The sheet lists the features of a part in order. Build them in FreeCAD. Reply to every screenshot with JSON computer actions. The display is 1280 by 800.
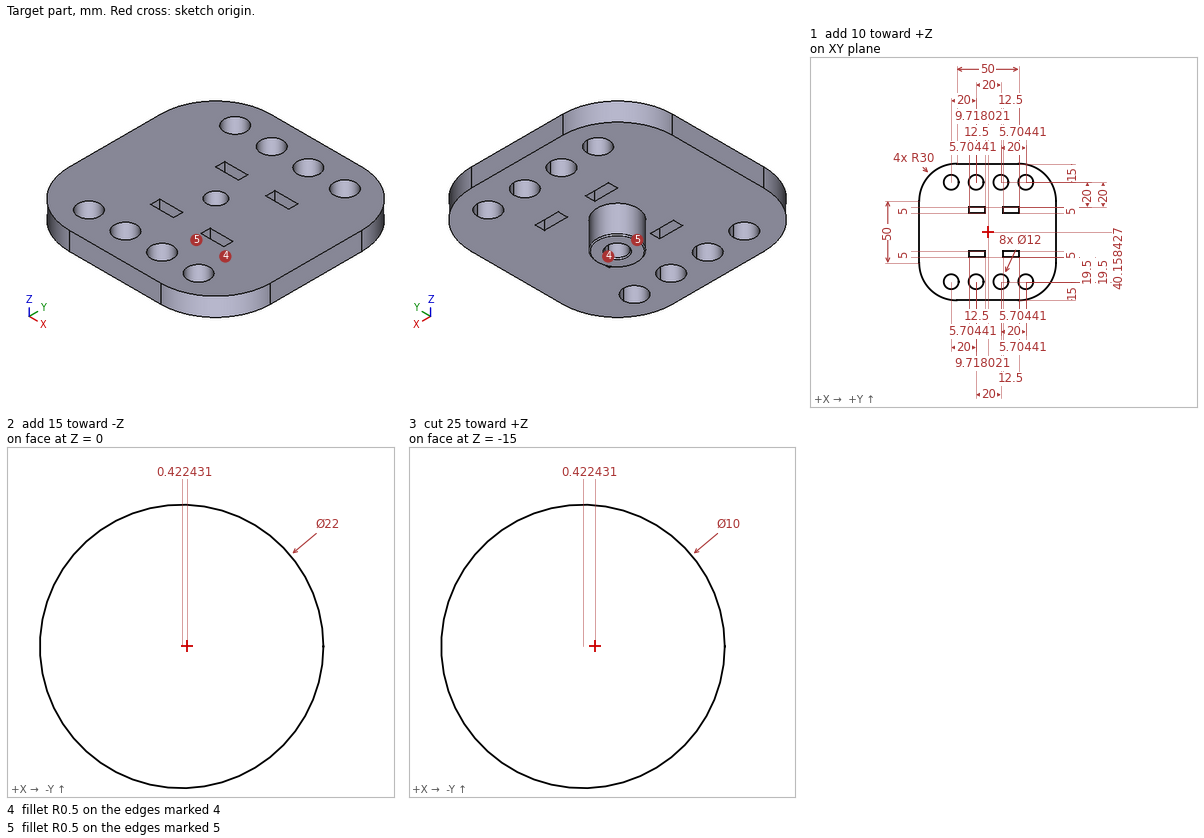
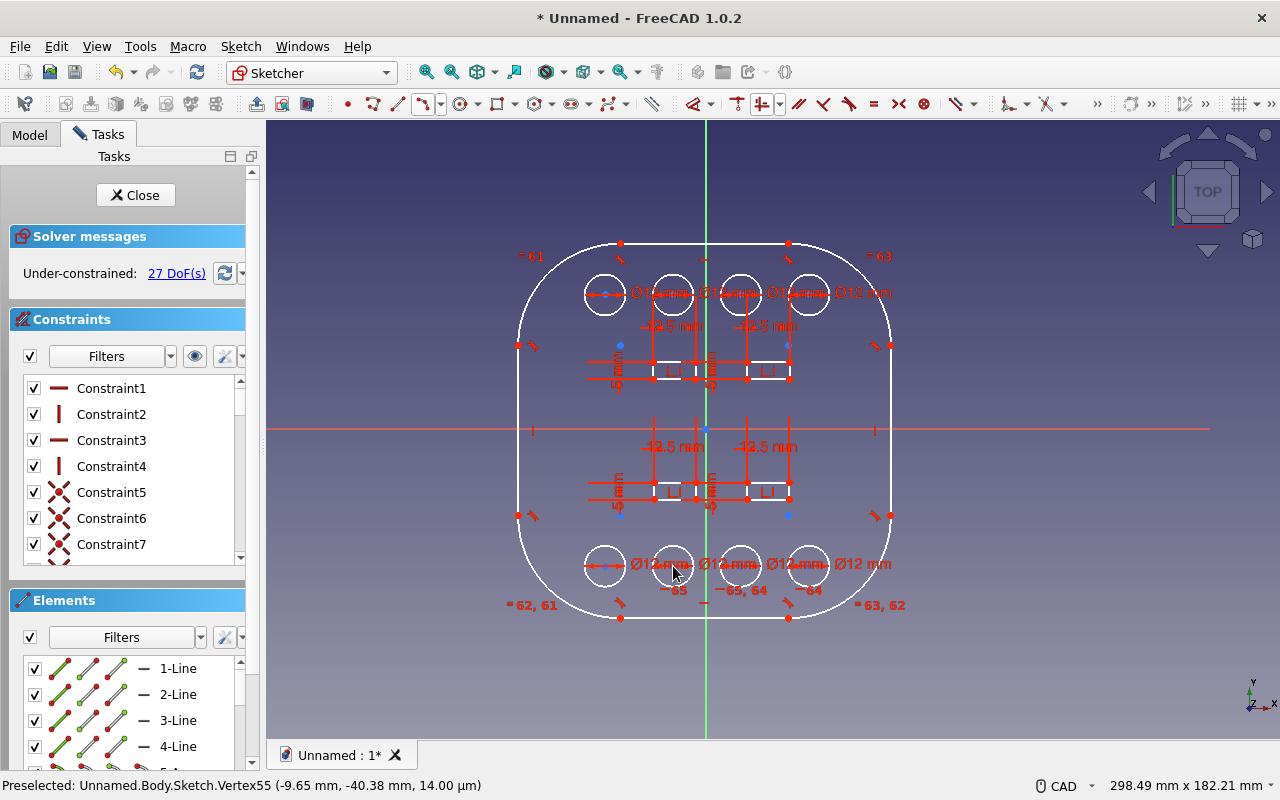
{"action": "left_click", "coordinate": [673, 566]}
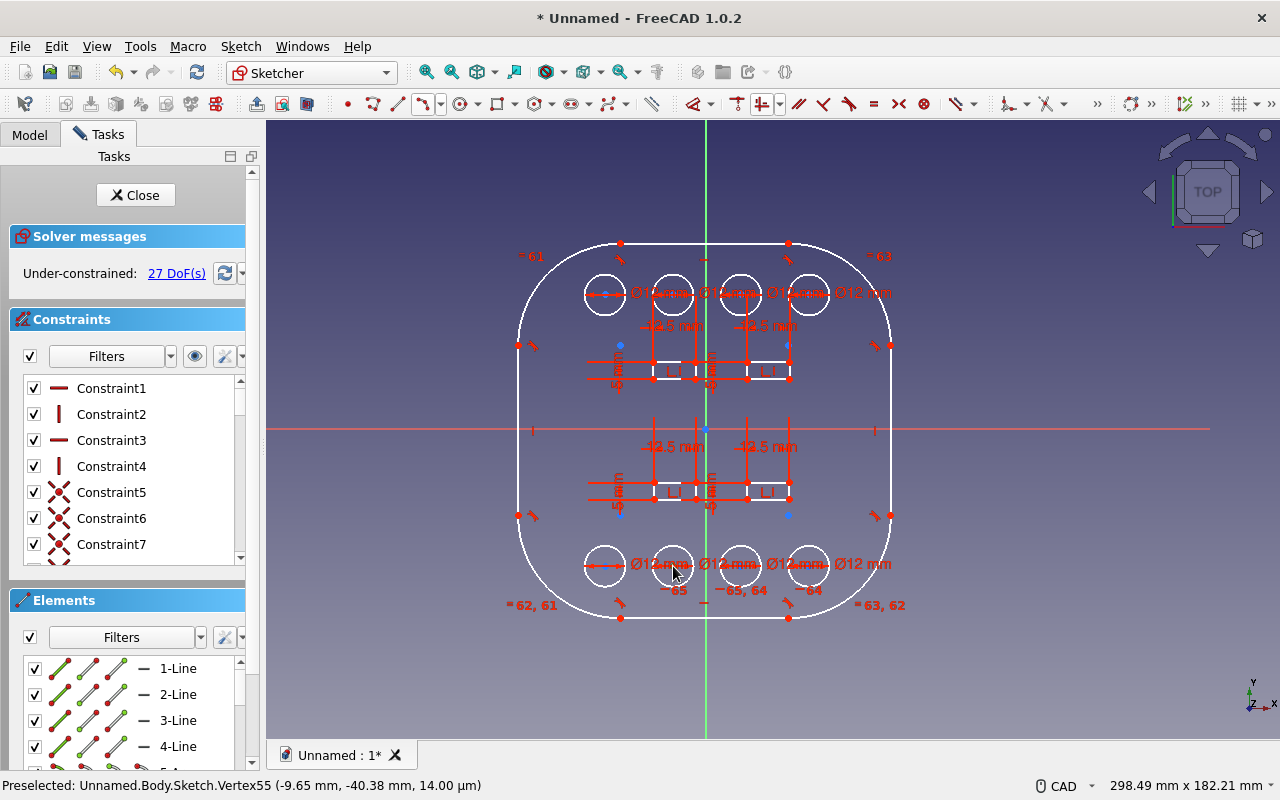
{"action": "left_click", "coordinate": [605, 566]}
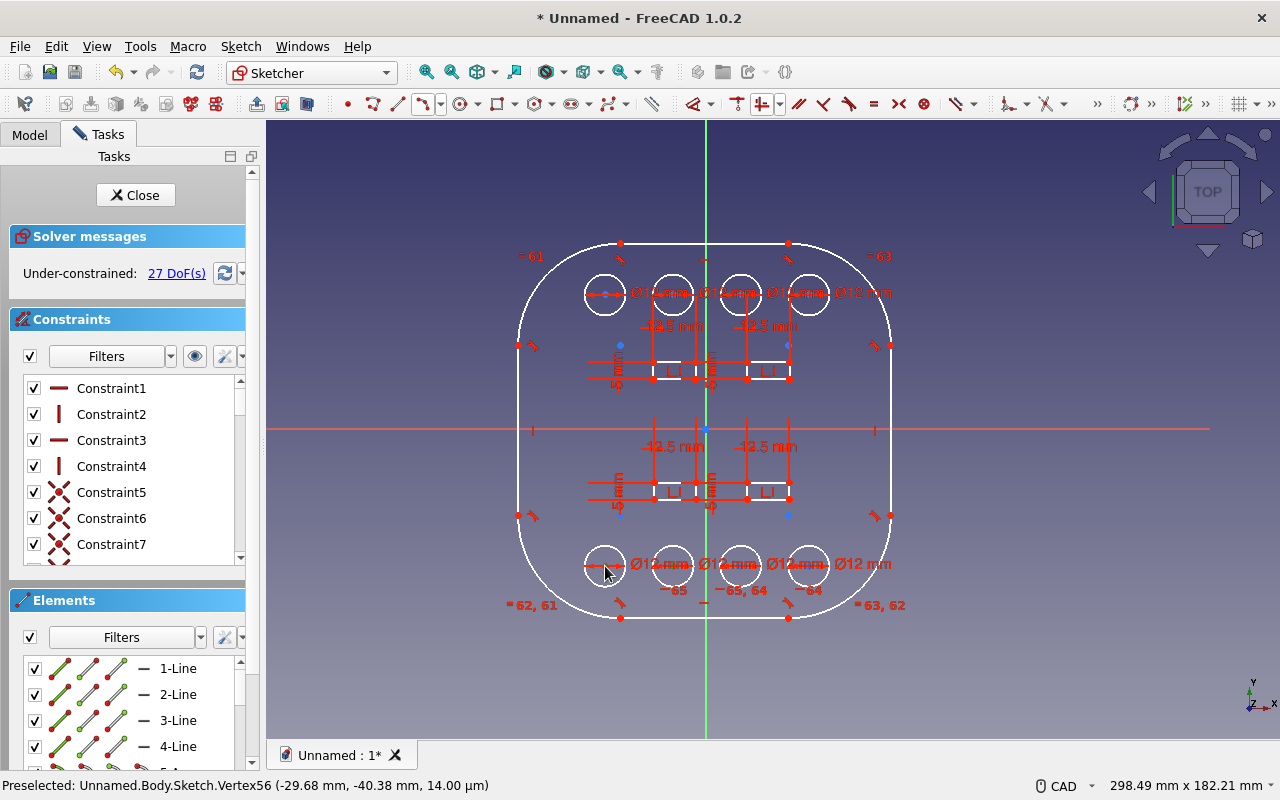
{"action": "key", "text": "h"}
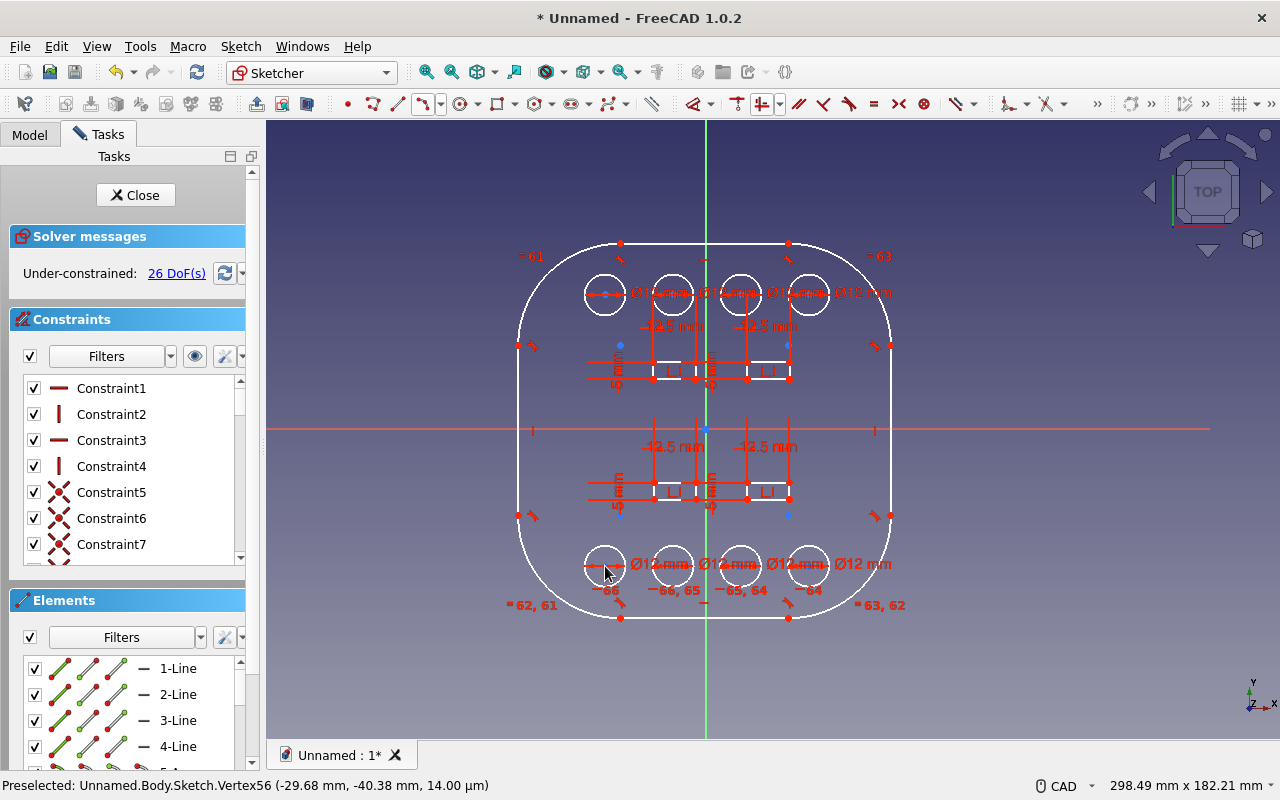
{"action": "left_click", "coordinate": [809, 295]}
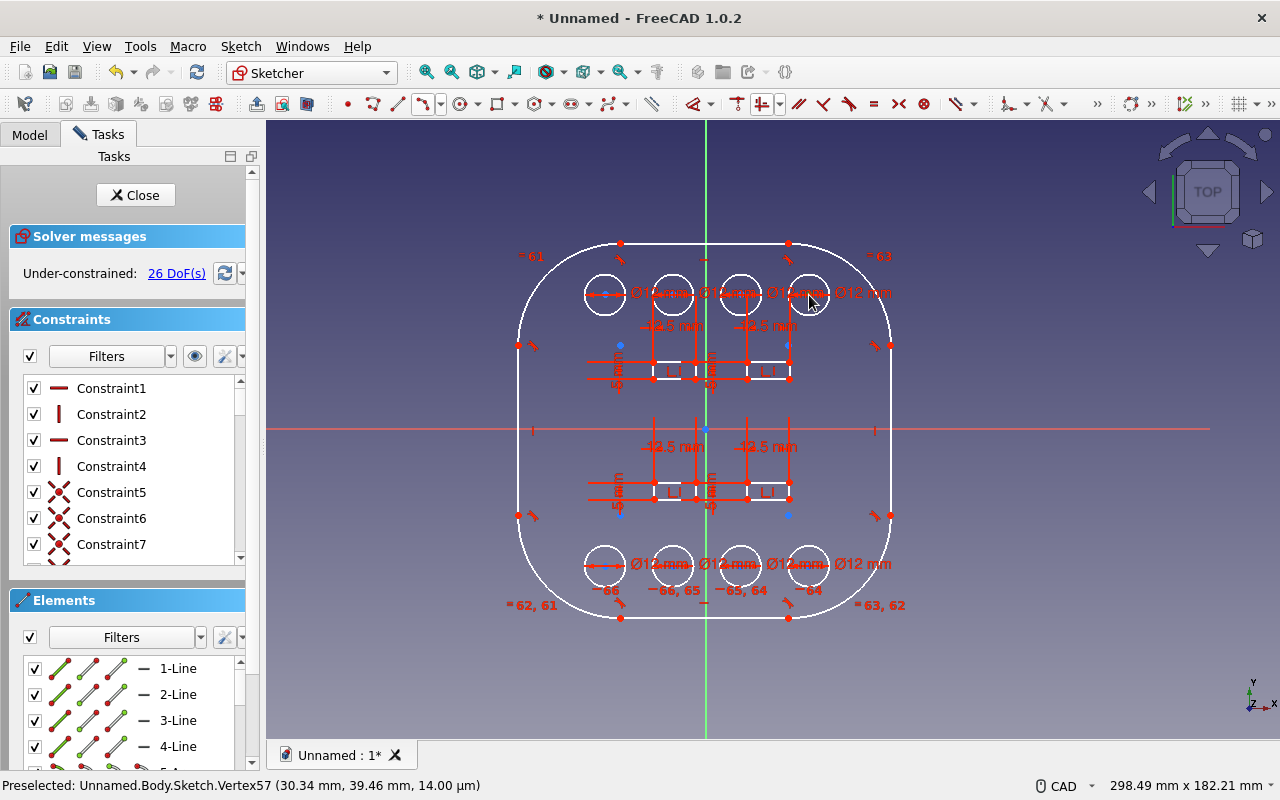
{"action": "left_click", "coordinate": [741, 295]}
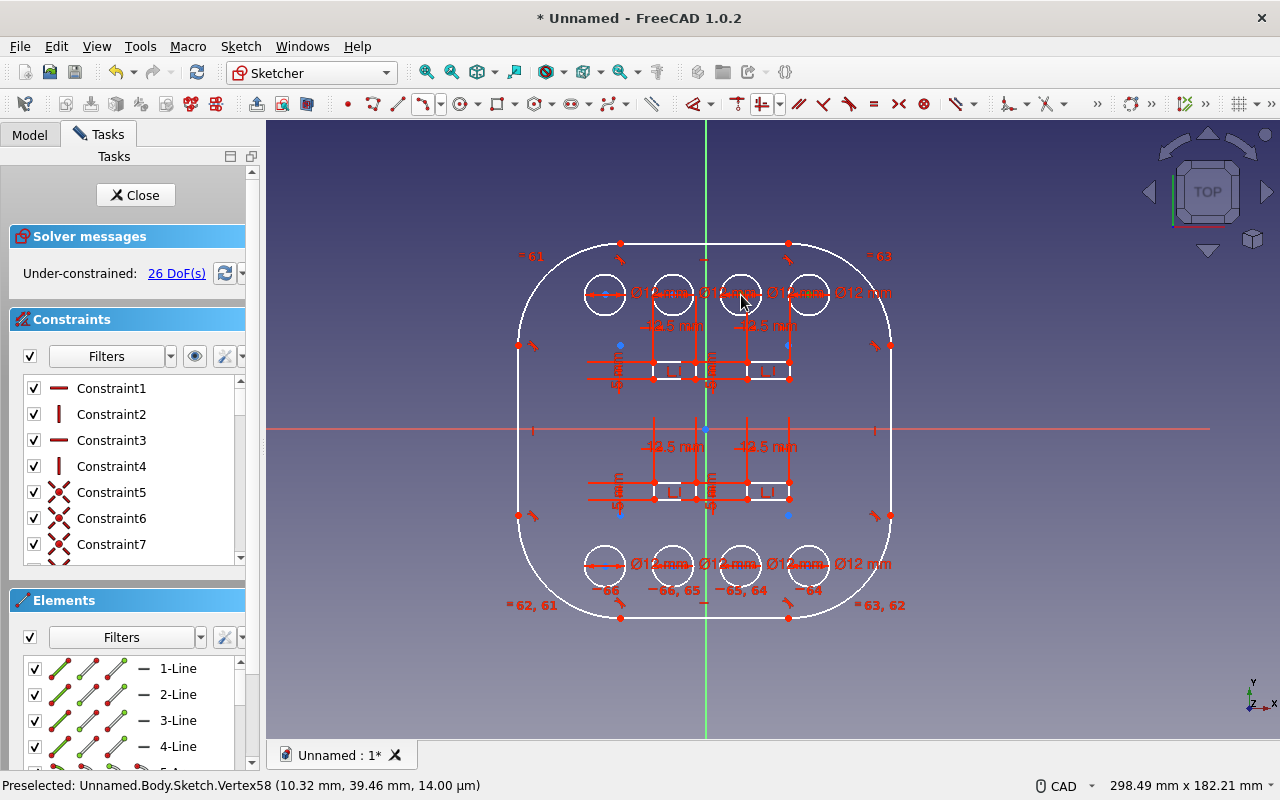
{"action": "left_click", "coordinate": [780, 104]}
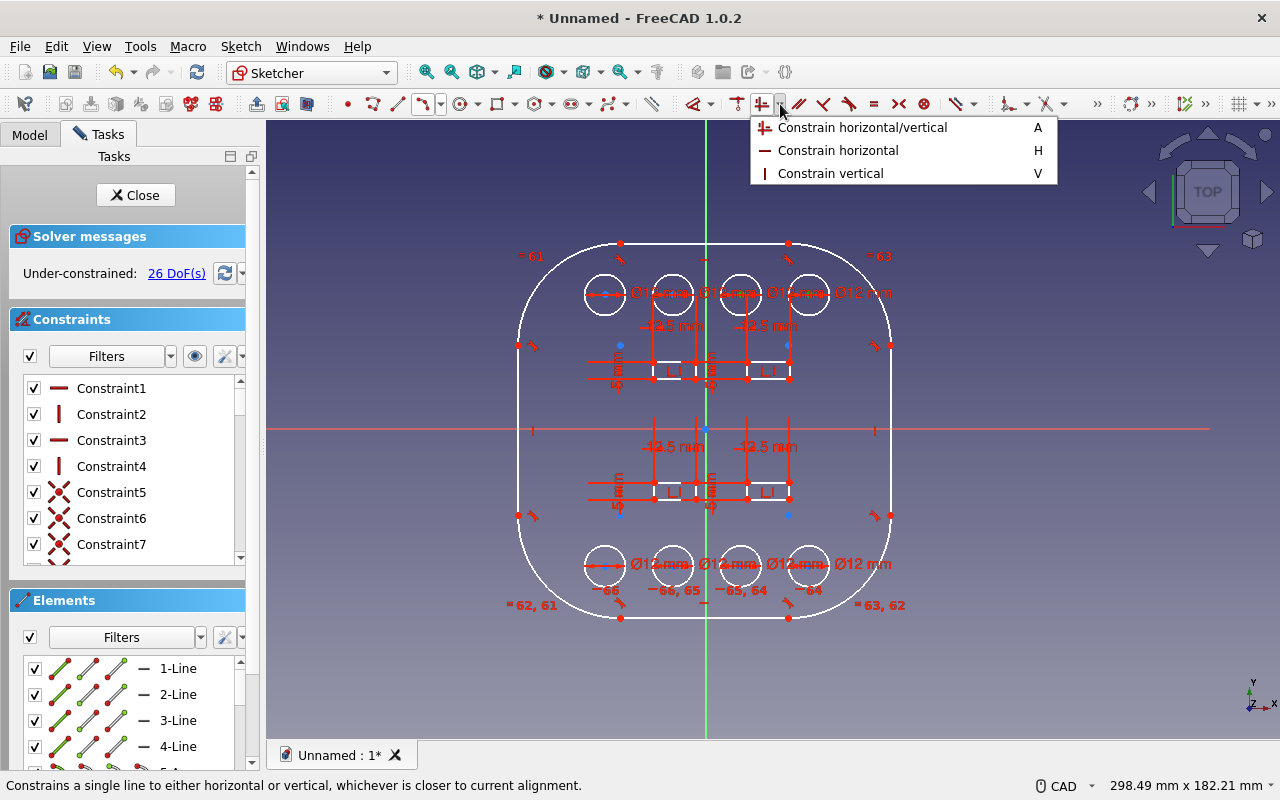
{"action": "left_click", "coordinate": [904, 150]}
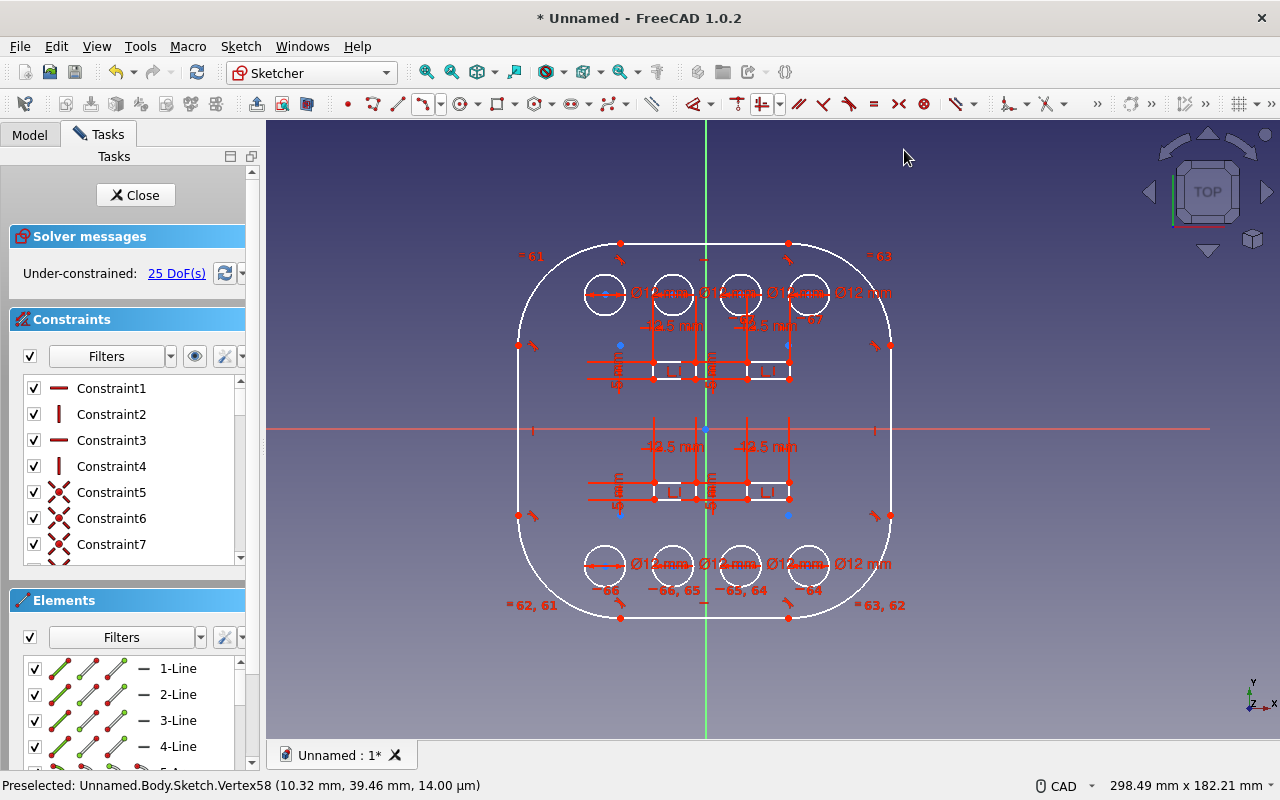
{"action": "left_click", "coordinate": [741, 295]}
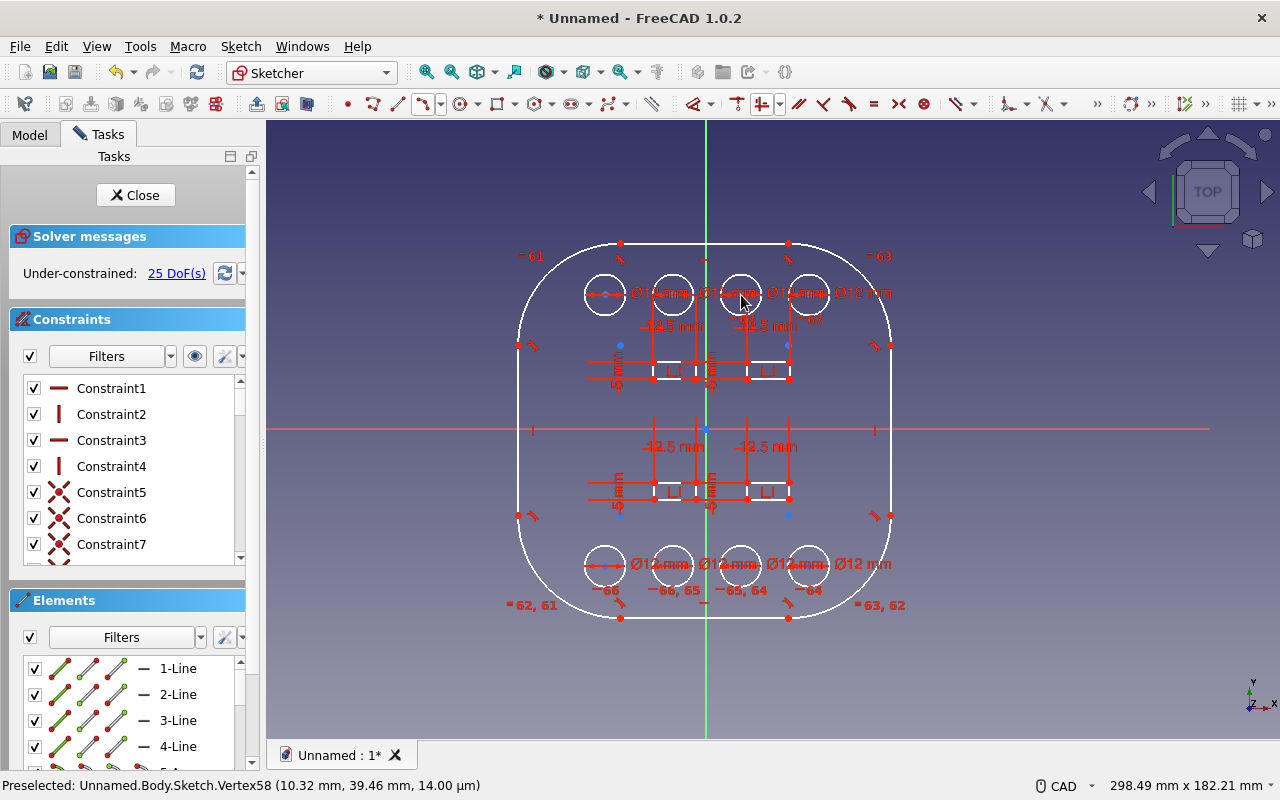
{"action": "left_click", "coordinate": [673, 295]}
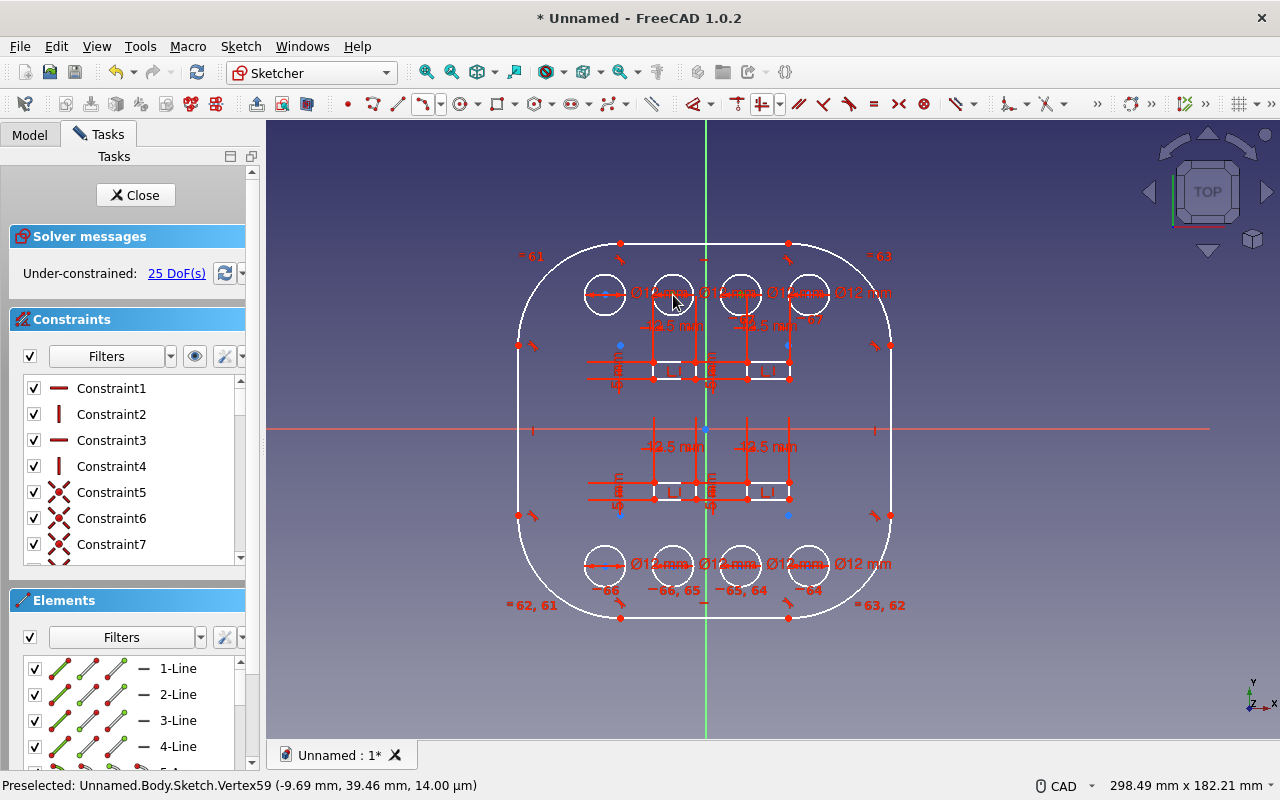
{"action": "left_click", "coordinate": [780, 104]}